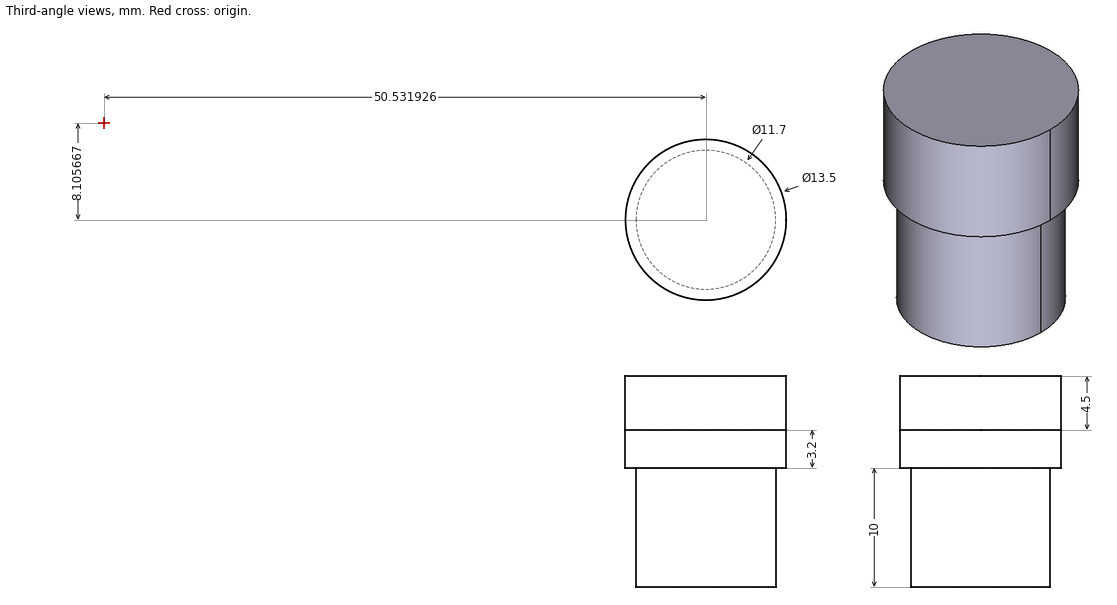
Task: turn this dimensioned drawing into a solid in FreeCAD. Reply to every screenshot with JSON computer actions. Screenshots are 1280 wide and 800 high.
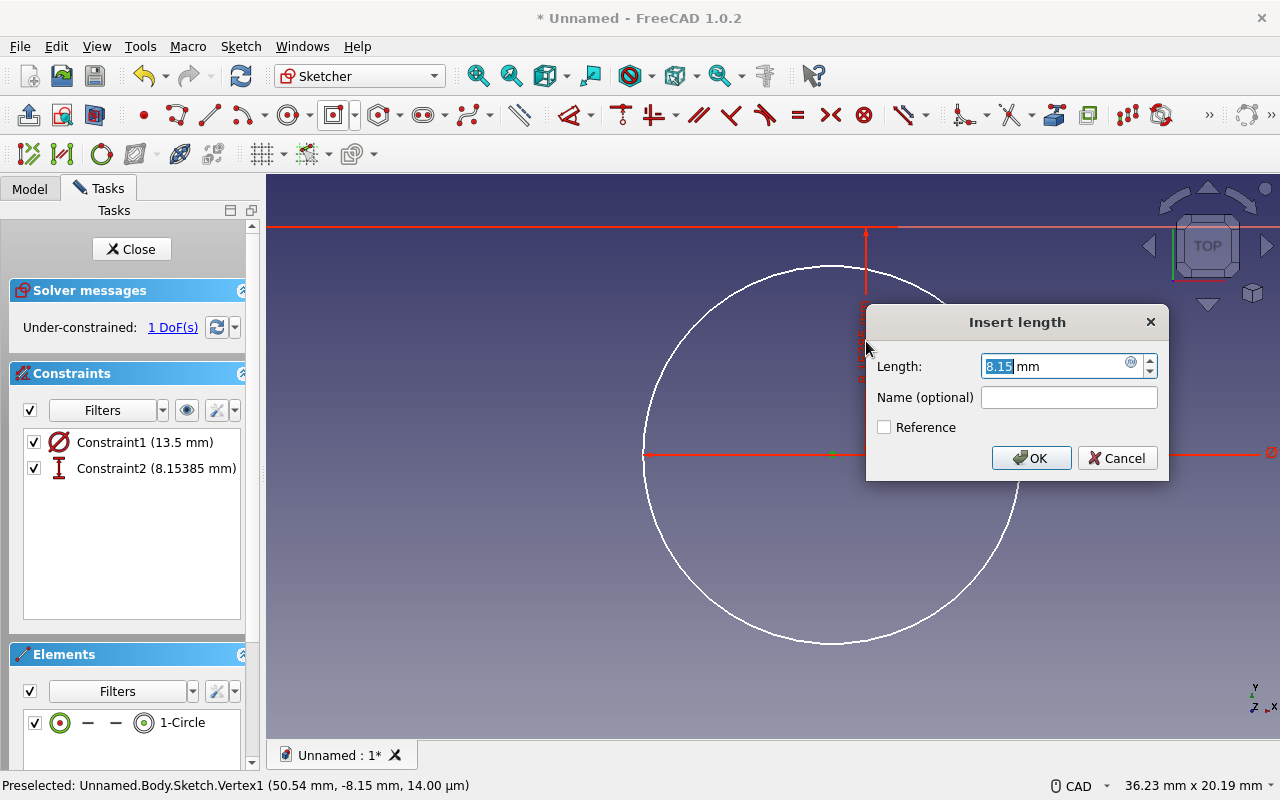
{"action": "type", "text": "8.105667"}
{"action": "key", "text": "Return"}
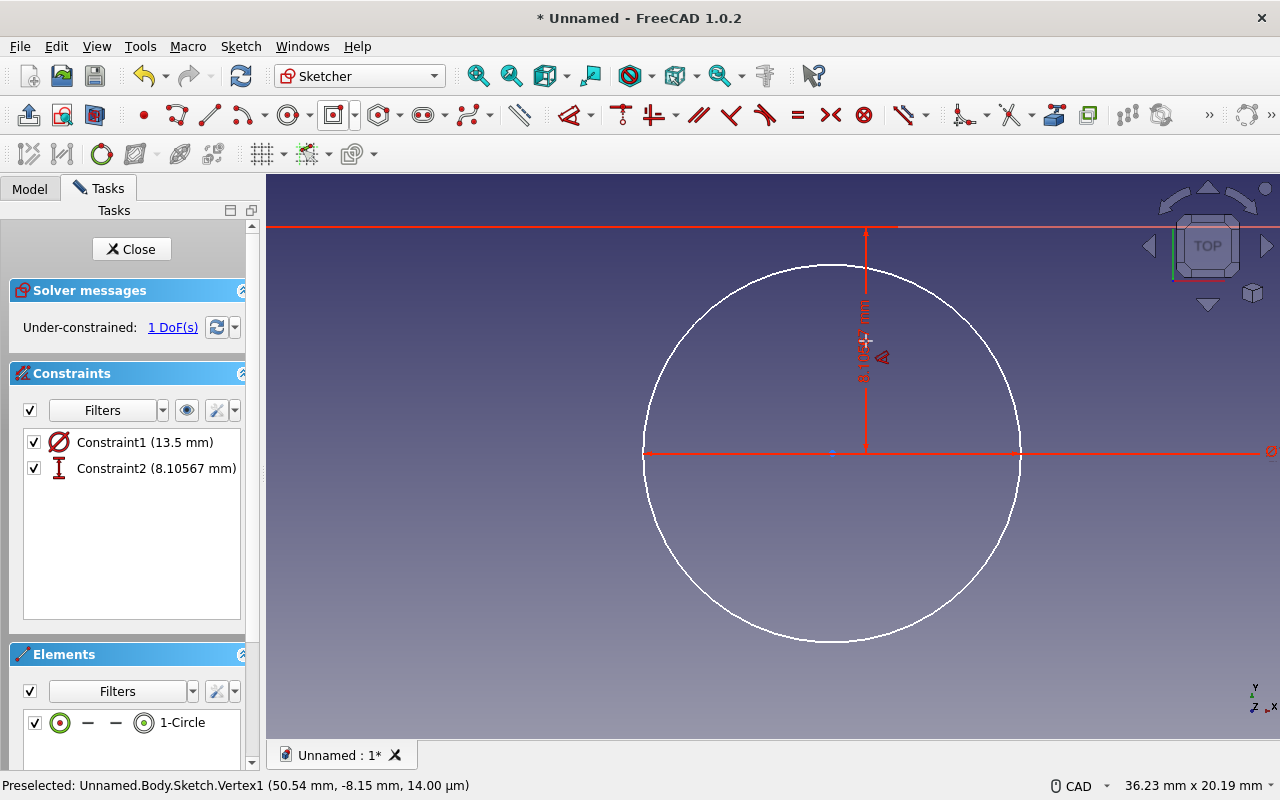
{"action": "left_click", "coordinate": [832, 454]}
{"action": "left_click", "coordinate": [563, 488]}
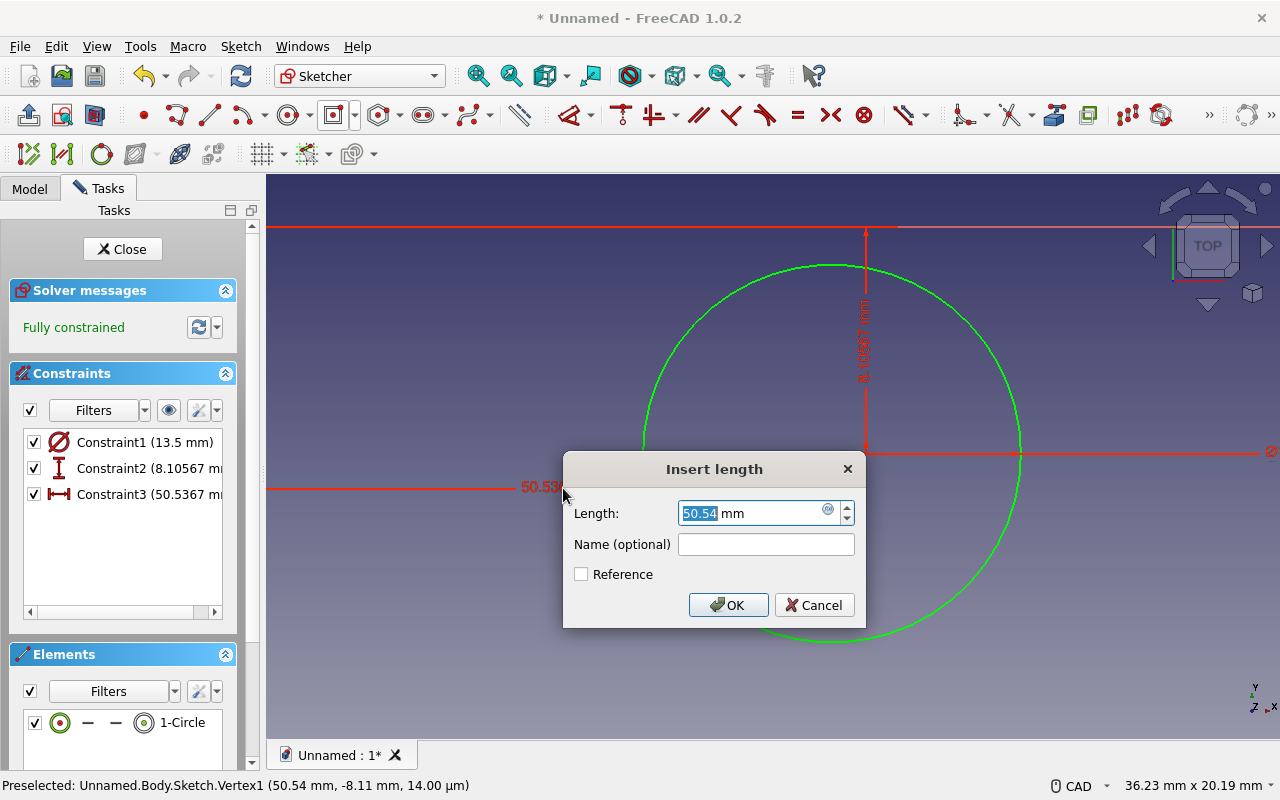
{"action": "type", "text": "50.531926"}
{"action": "key", "text": "Return"}
{"action": "key", "text": "Escape"}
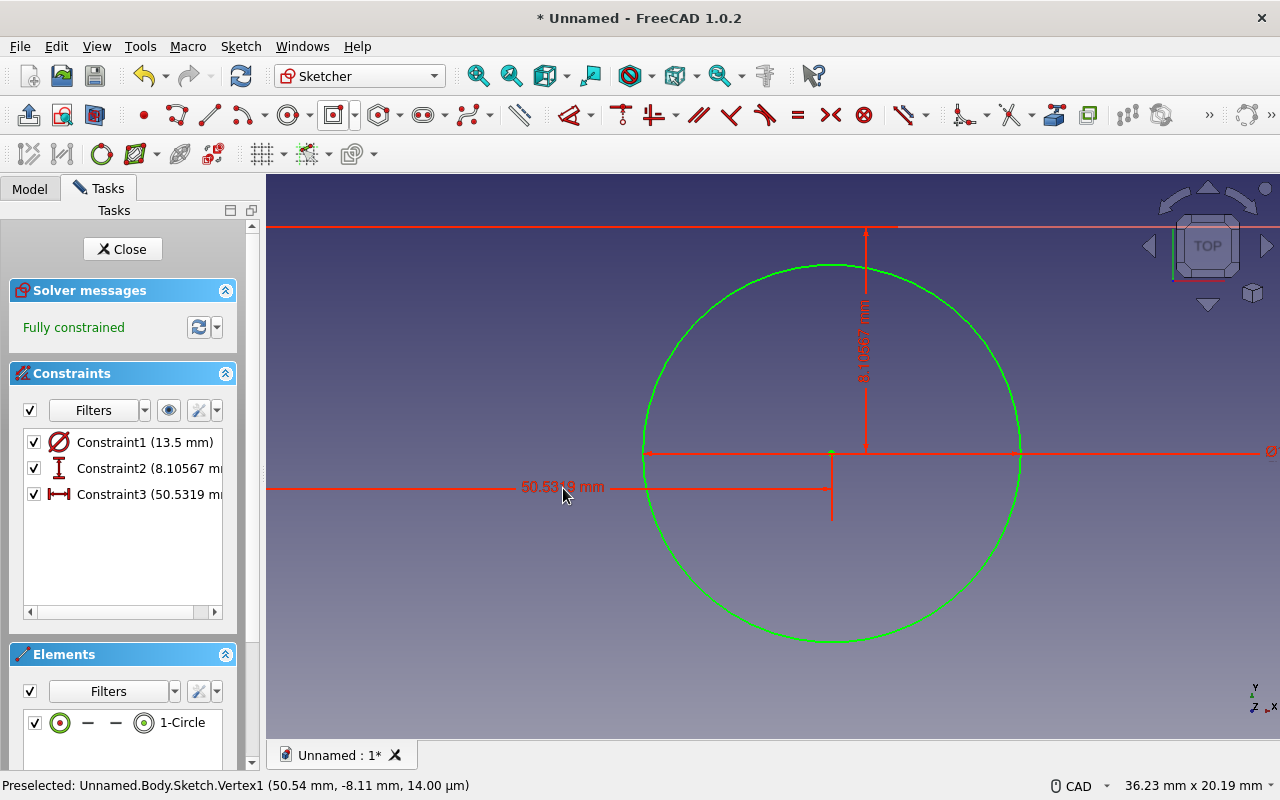
{"action": "left_click", "coordinate": [123, 249]}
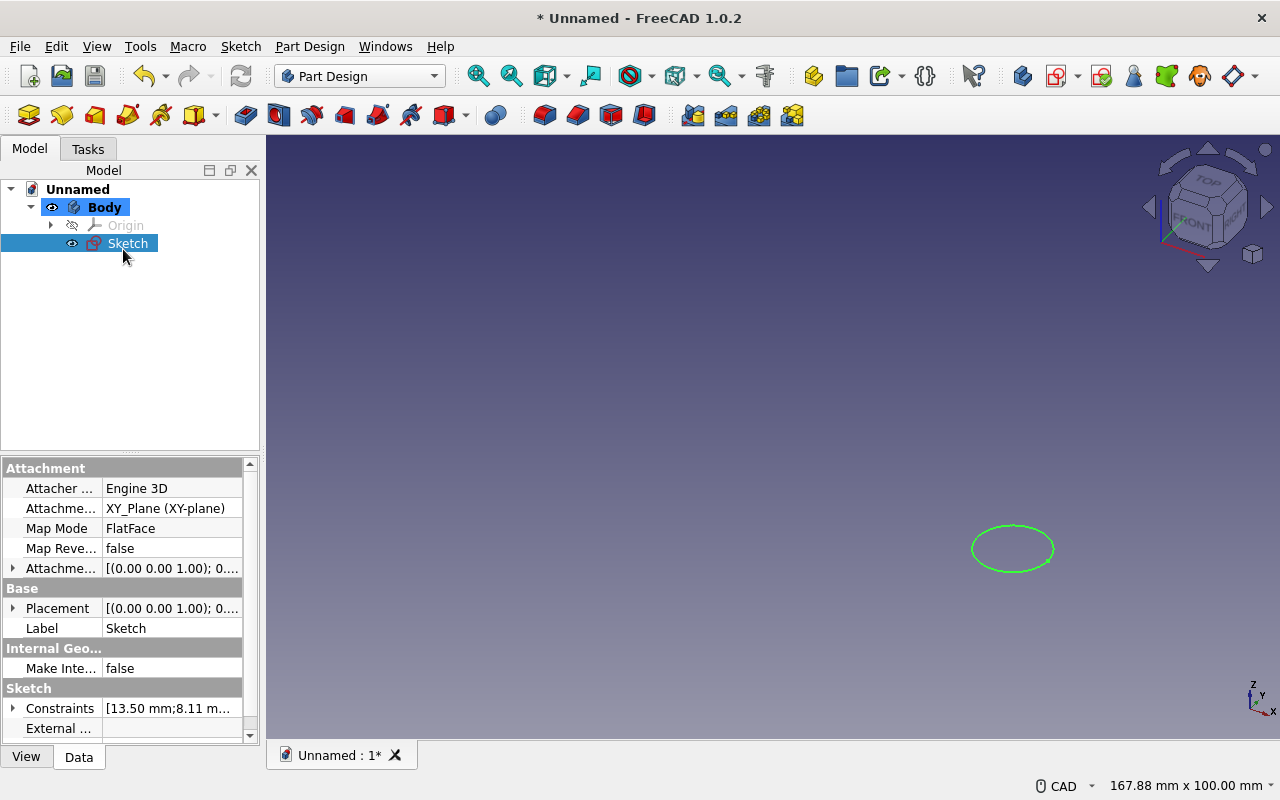
{"action": "left_click", "coordinate": [29, 116]}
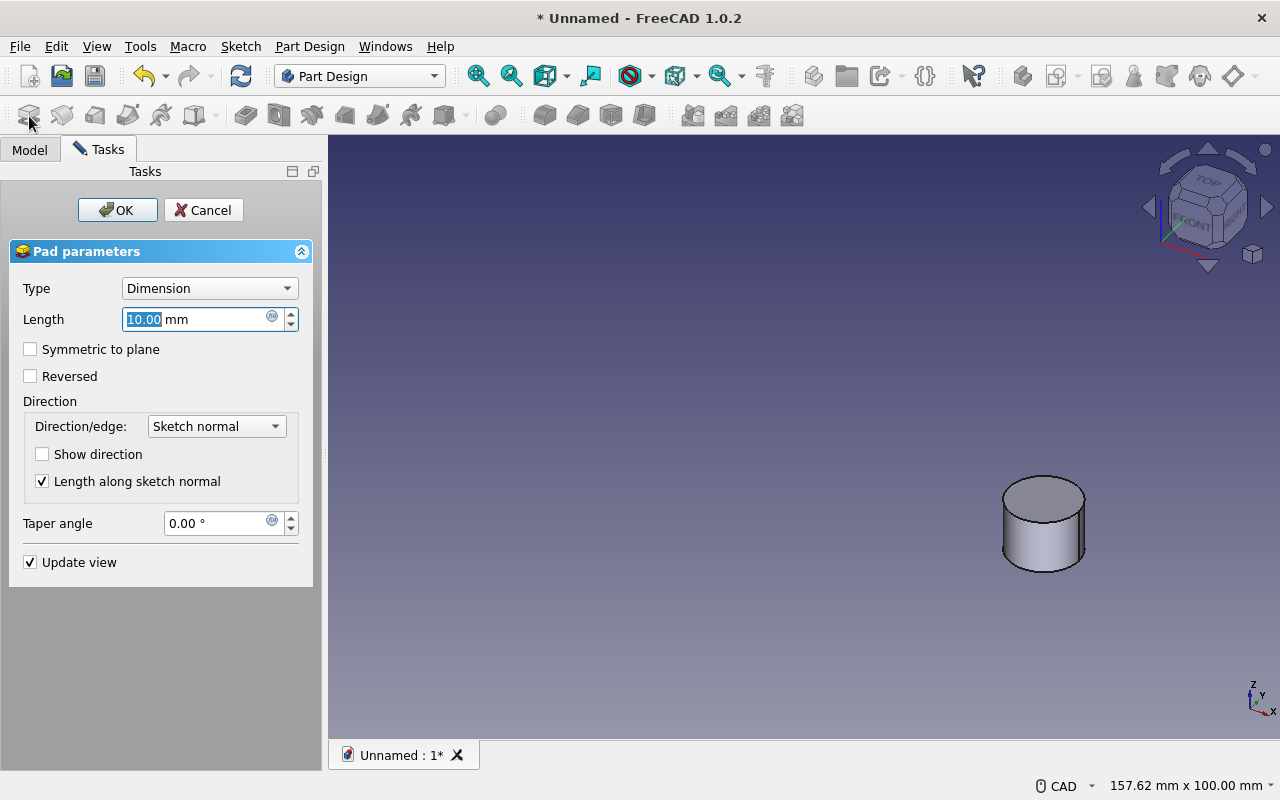
{"action": "type", "text": "4.5"}
{"action": "key", "text": "Tab"}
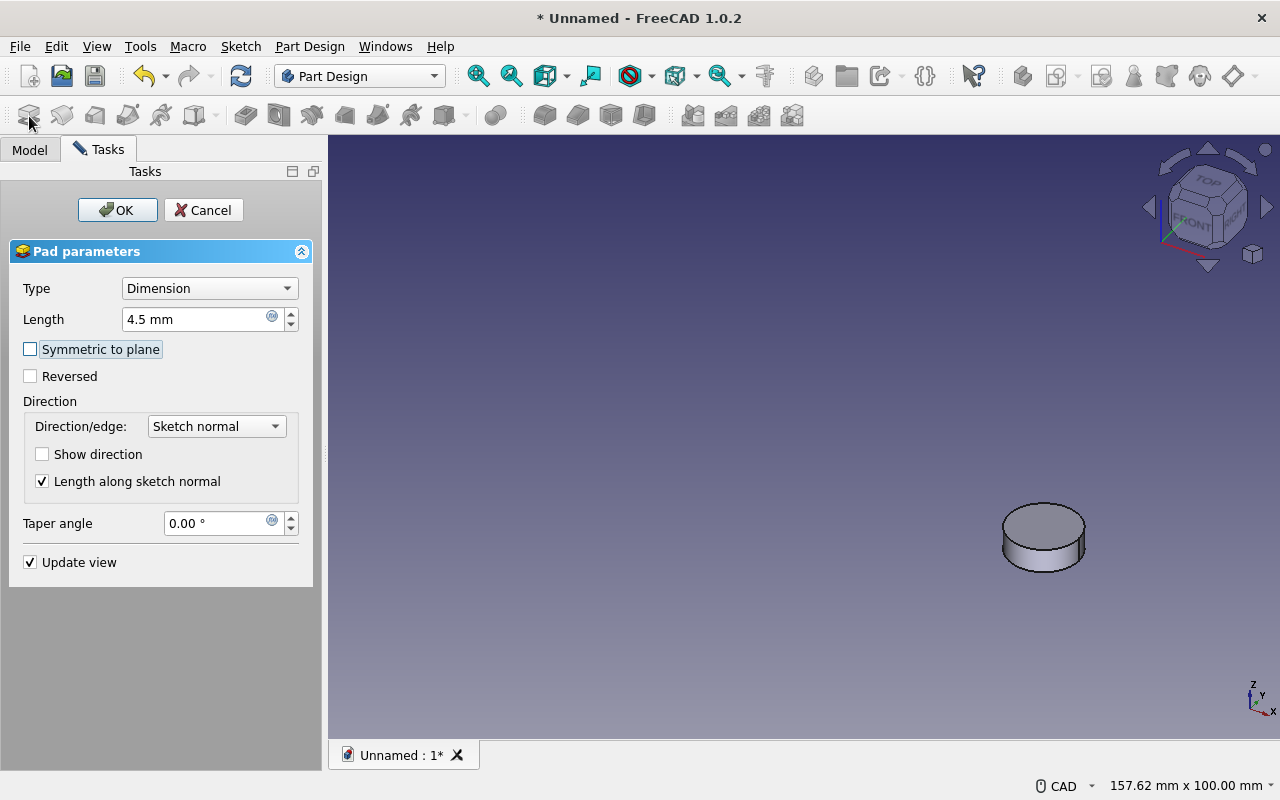
{"action": "left_click", "coordinate": [118, 210]}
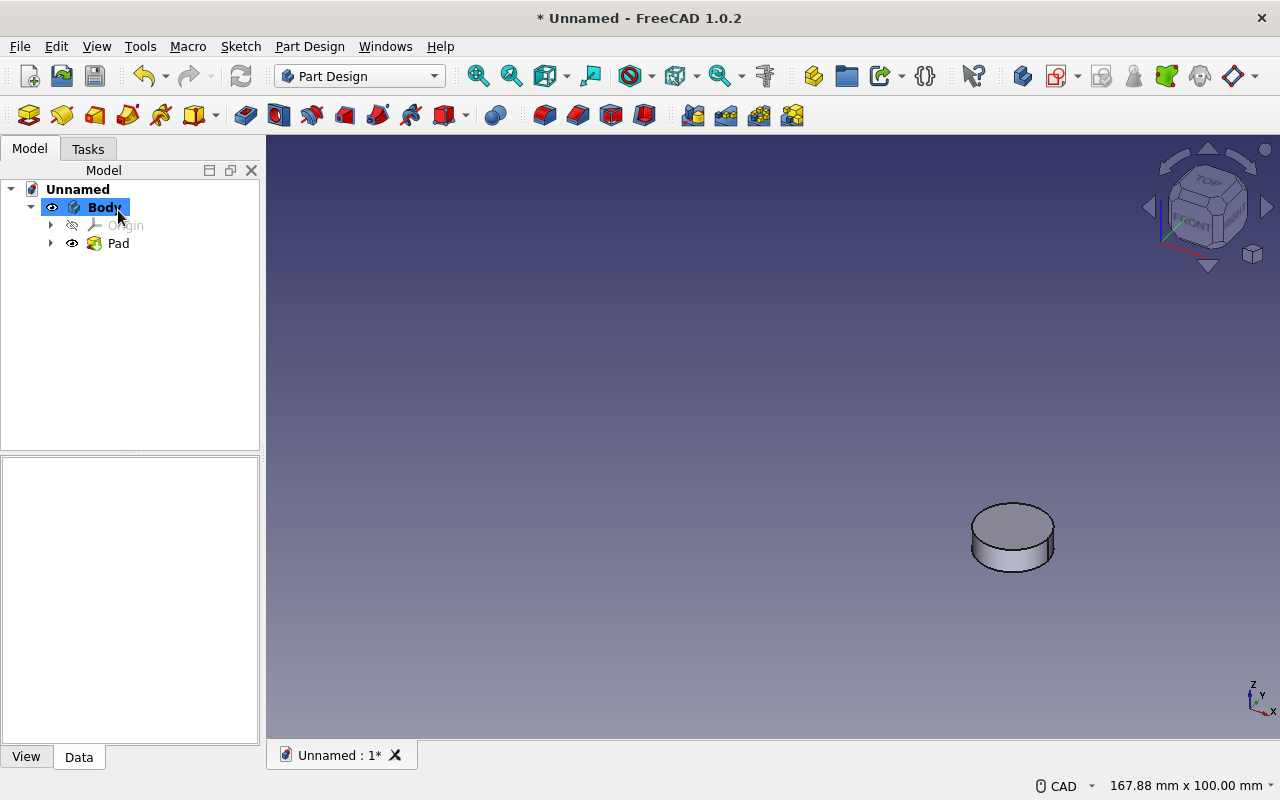
{"action": "key", "text": "v f"}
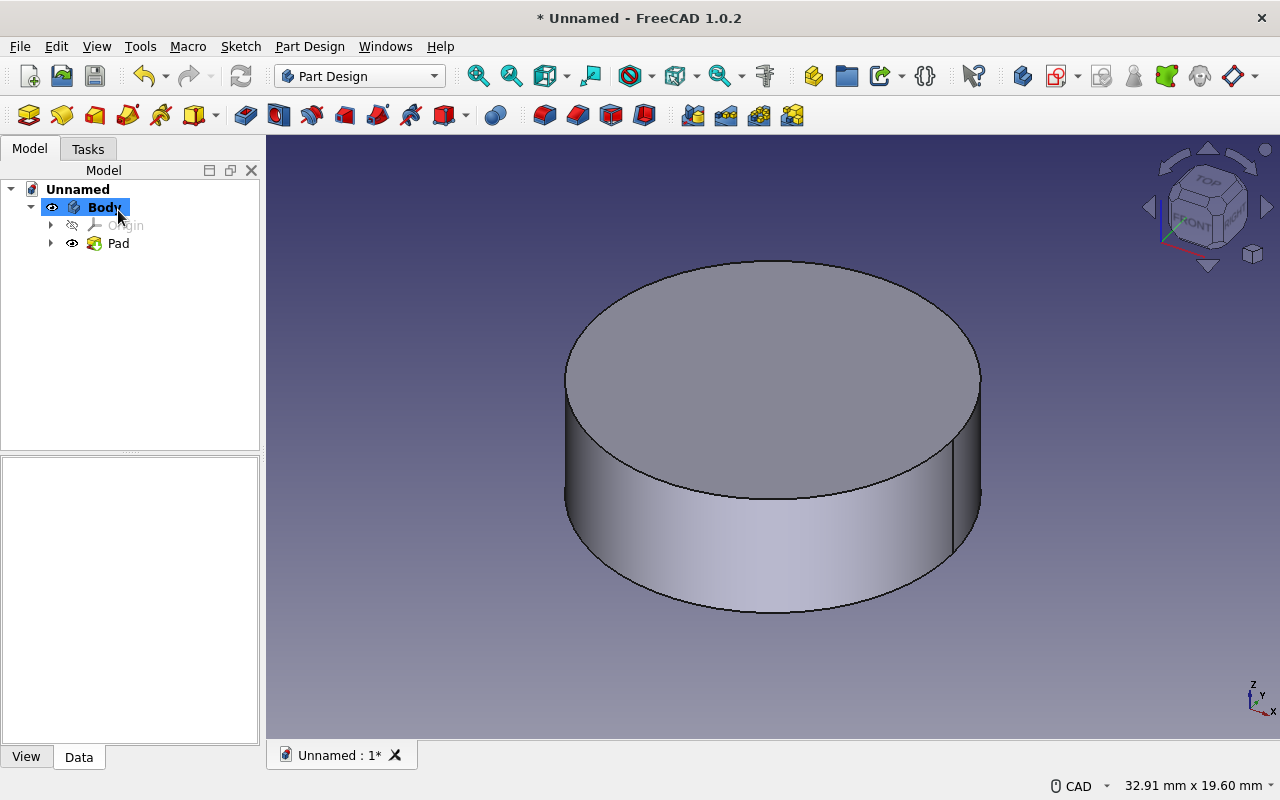
{"action": "left_click", "coordinate": [51, 225]}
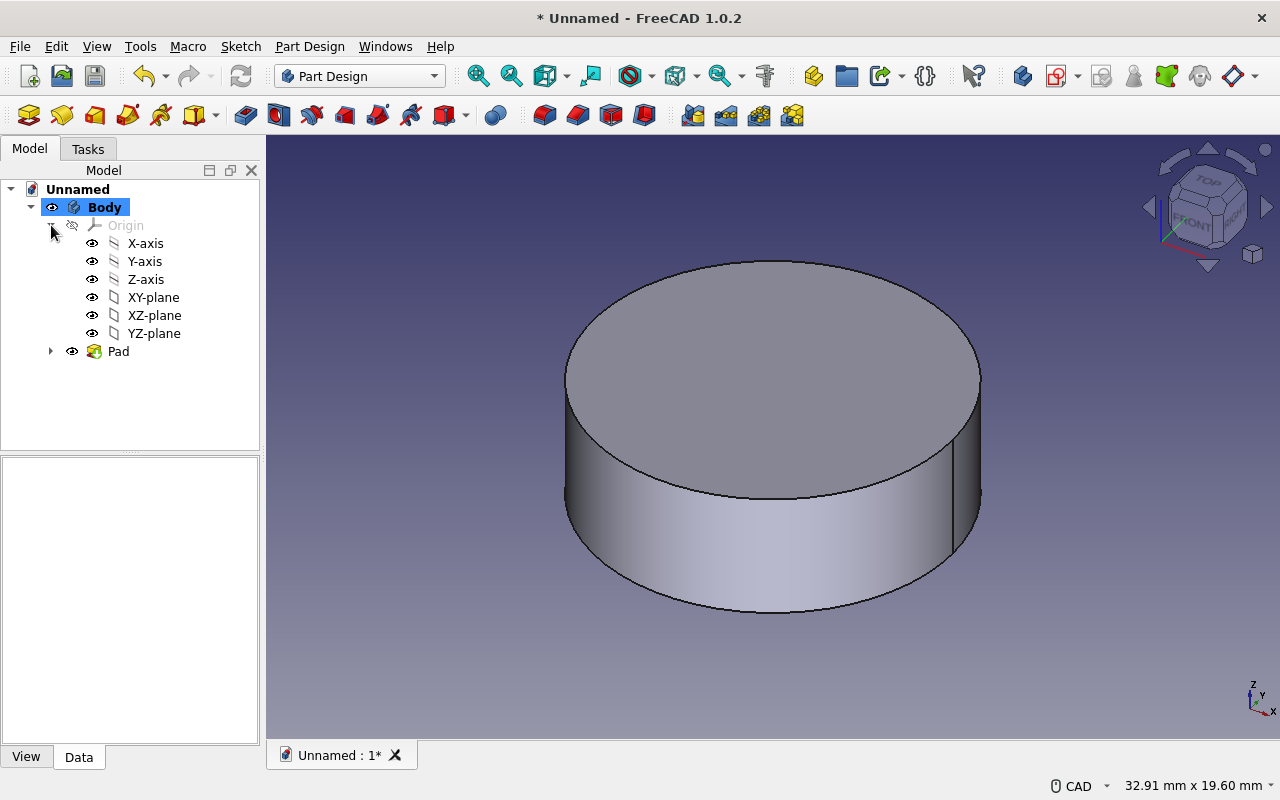
{"action": "left_click", "coordinate": [137, 297]}